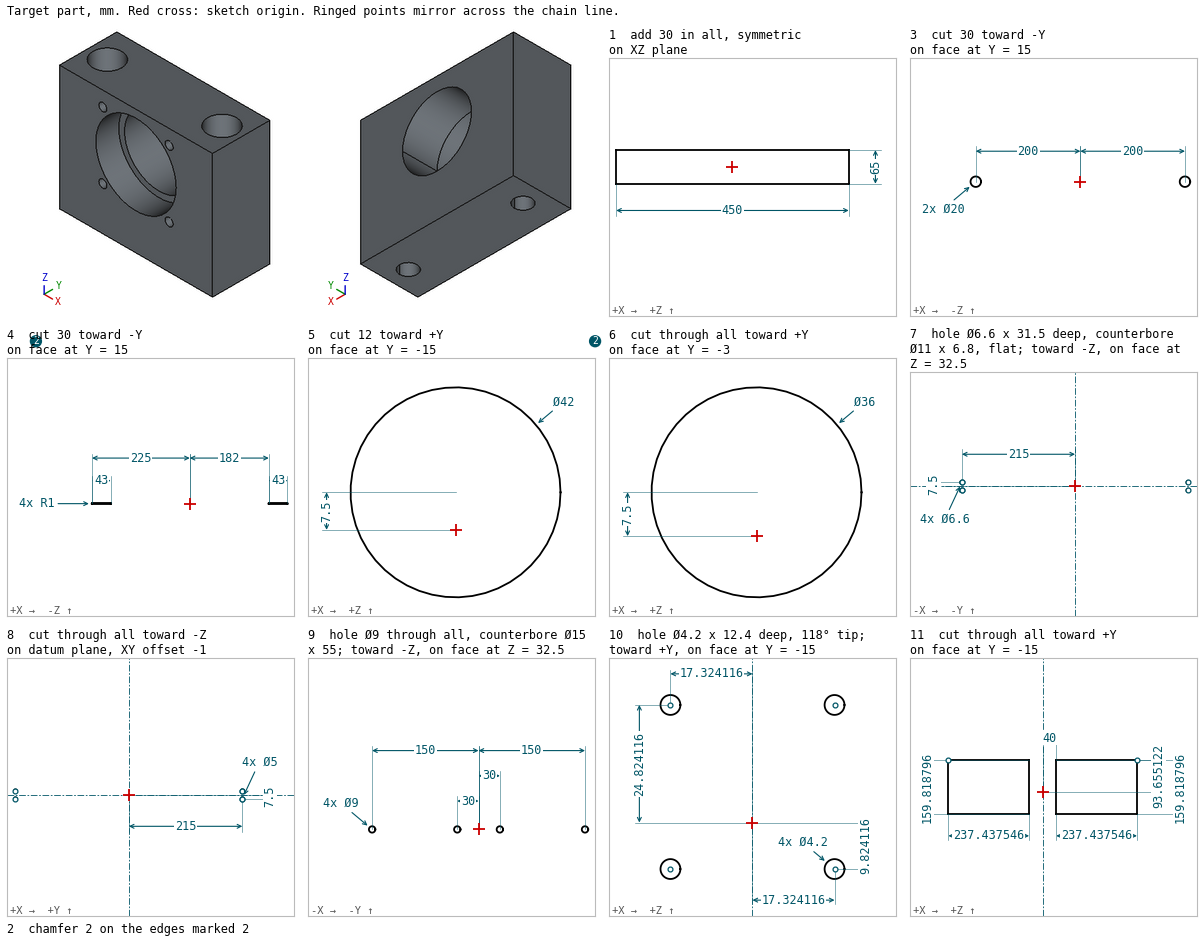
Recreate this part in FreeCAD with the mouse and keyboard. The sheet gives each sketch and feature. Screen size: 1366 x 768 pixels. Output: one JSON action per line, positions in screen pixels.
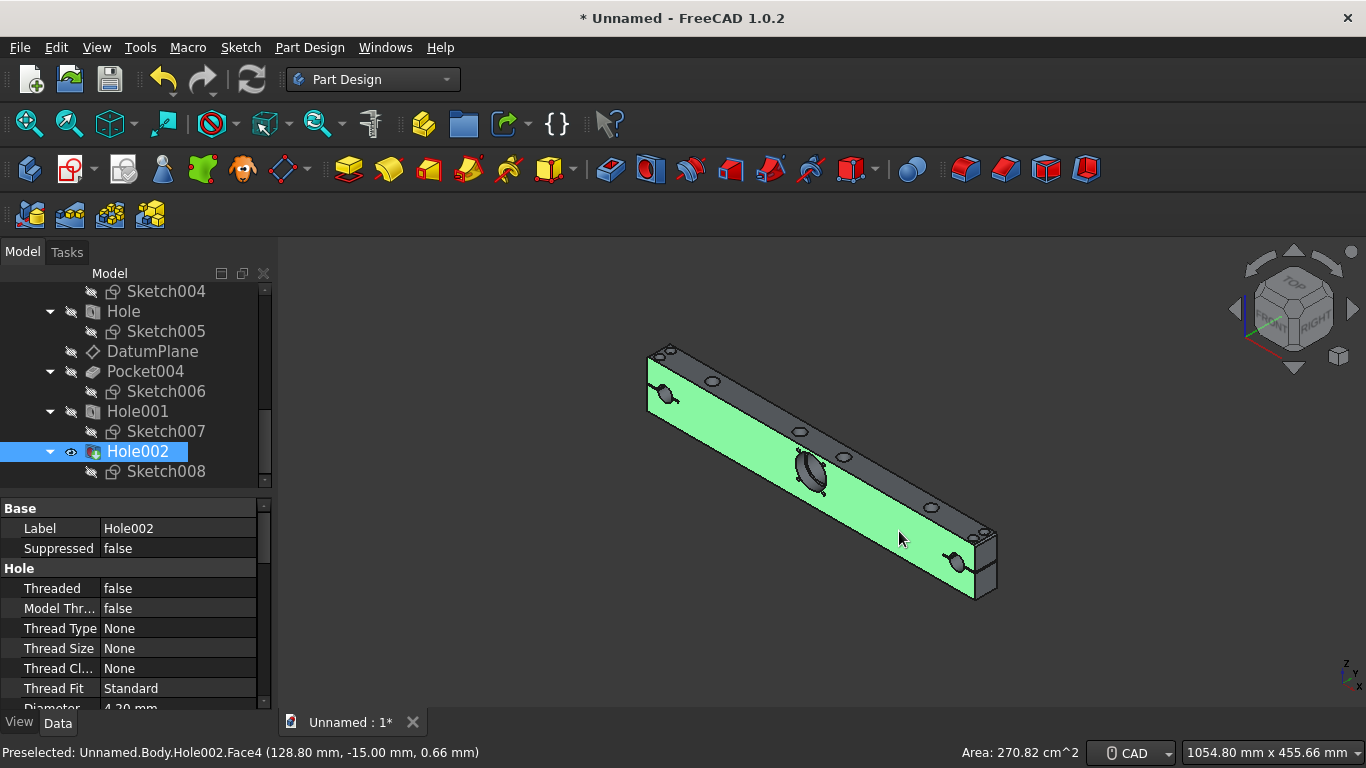
{"action": "left_click", "coordinate": [70, 170]}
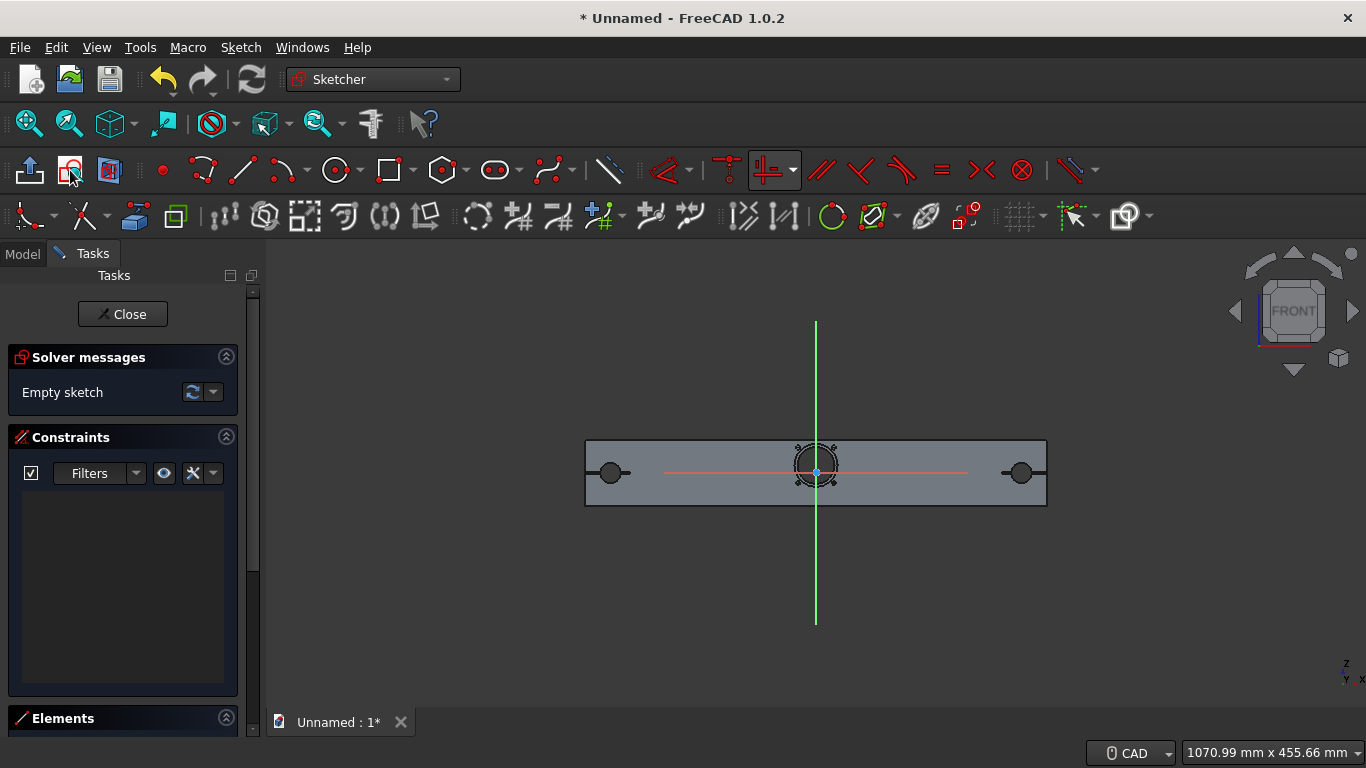
{"action": "key", "text": "g r"}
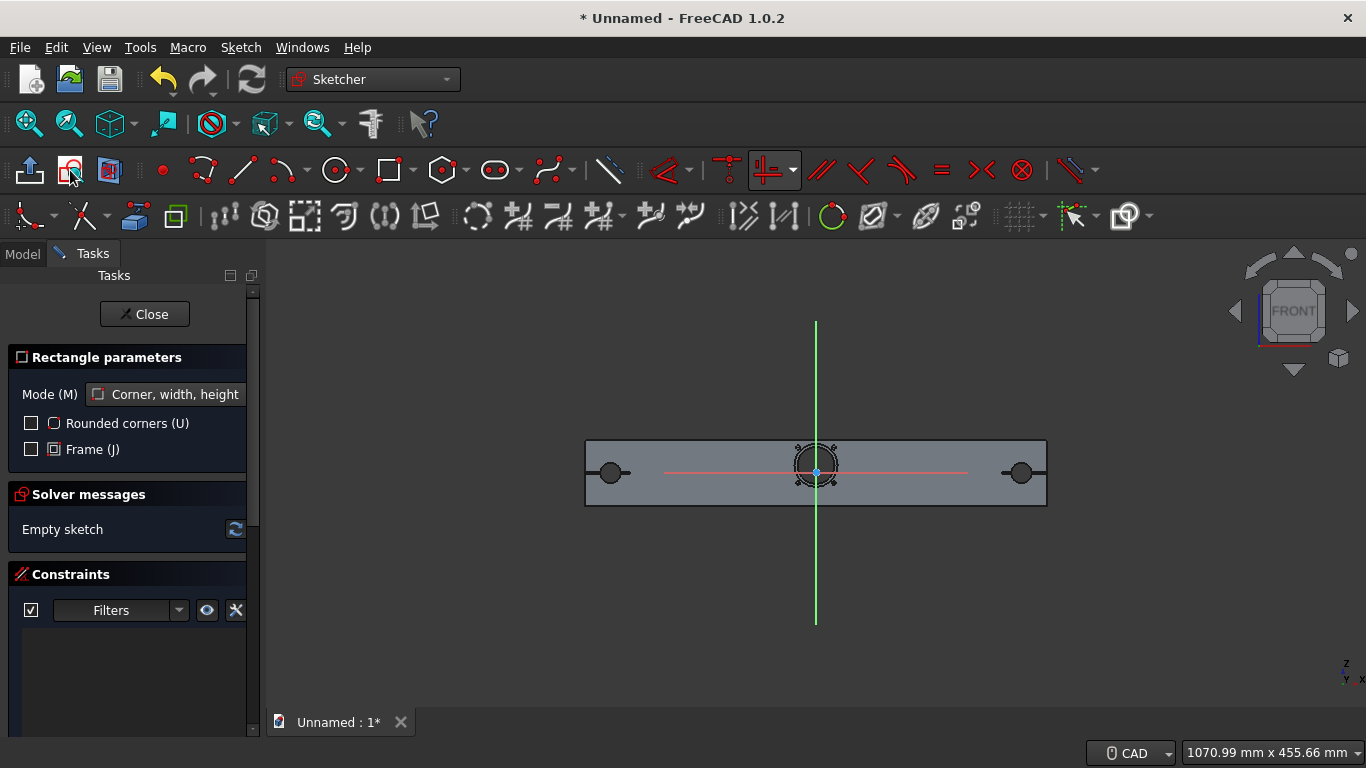
{"action": "left_click", "coordinate": [857, 377]}
{"action": "mouse_move", "coordinate": [1101, 541]}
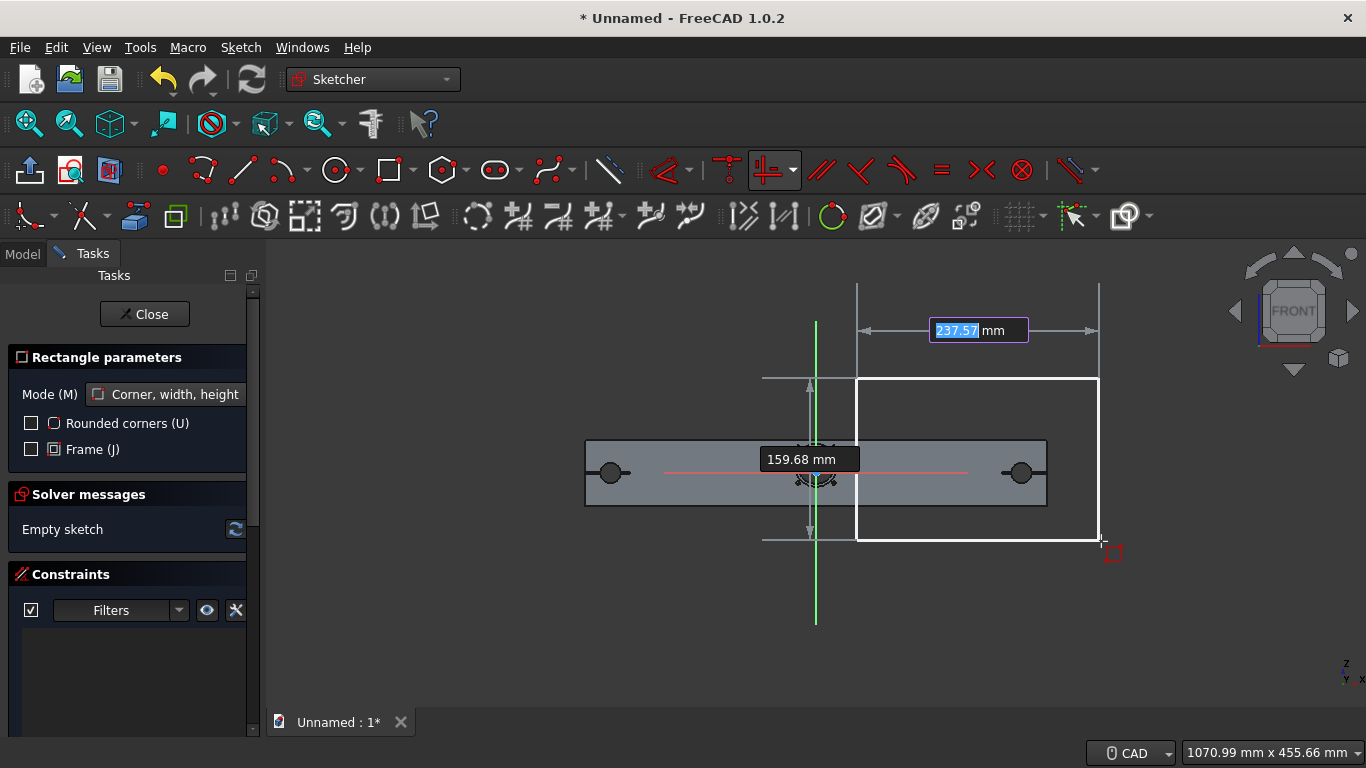
{"action": "type", "text": "237.437546"}
{"action": "key", "text": "Tab"}
{"action": "type", "text": "159.818796"}
{"action": "key", "text": "Return"}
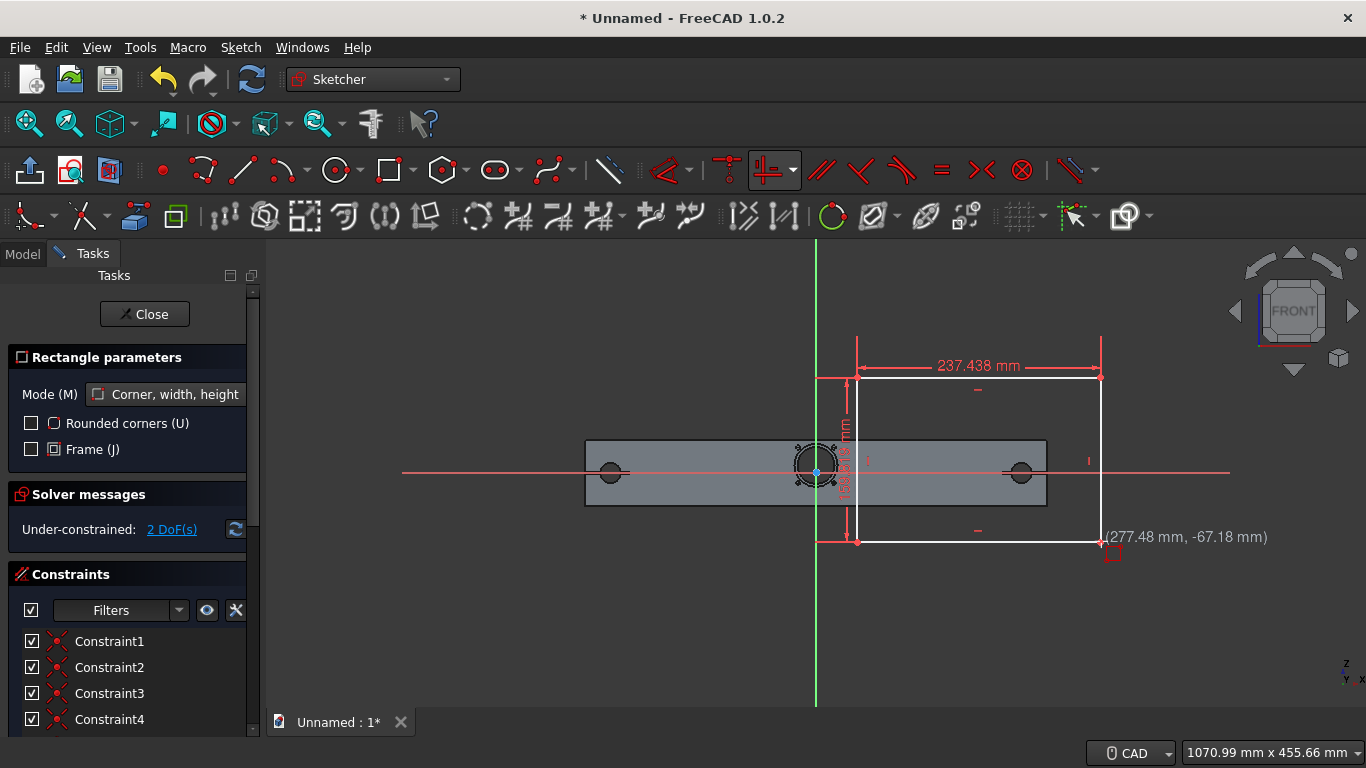
{"action": "left_click", "coordinate": [531, 377]}
{"action": "mouse_move", "coordinate": [775, 541]}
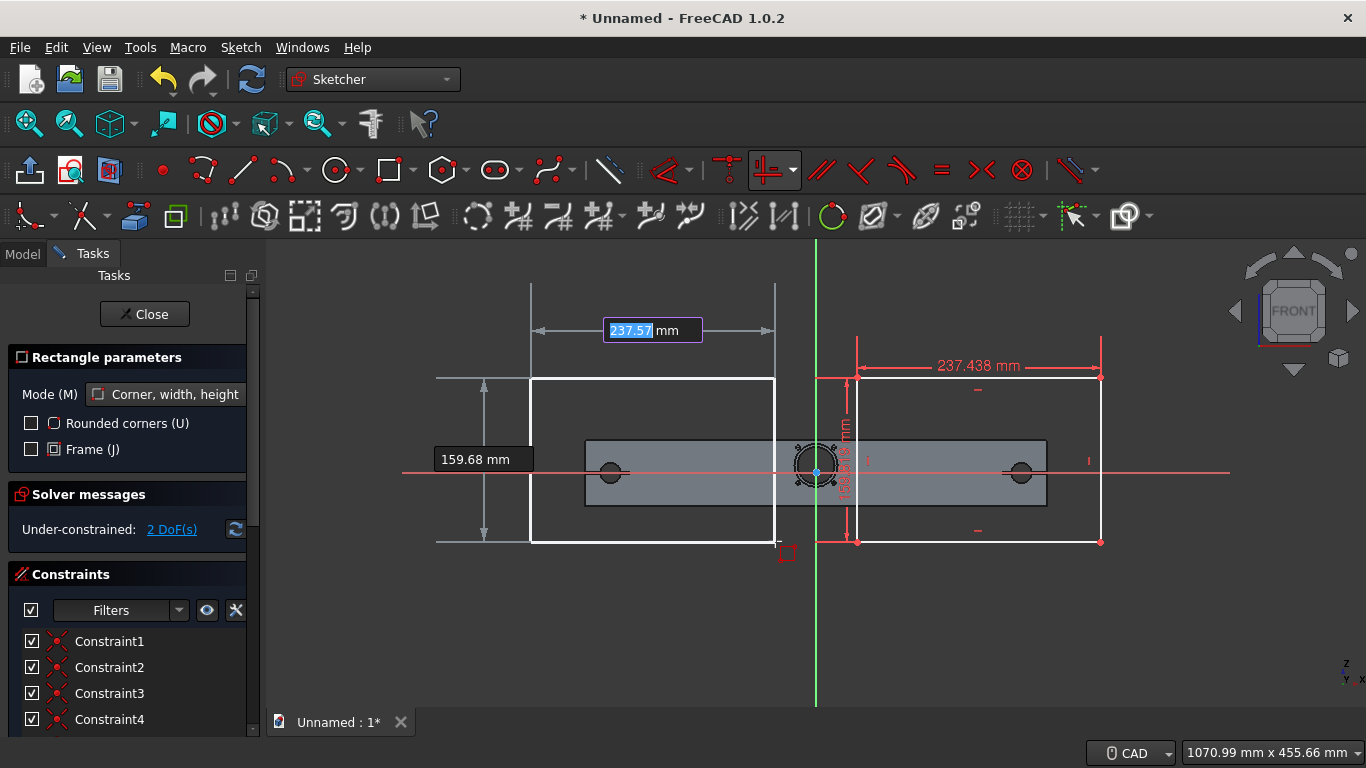
{"action": "type", "text": "237.437546"}
{"action": "key", "text": "Tab"}
{"action": "type", "text": "159.818796"}
{"action": "key", "text": "Return"}
{"action": "key", "text": "Escape"}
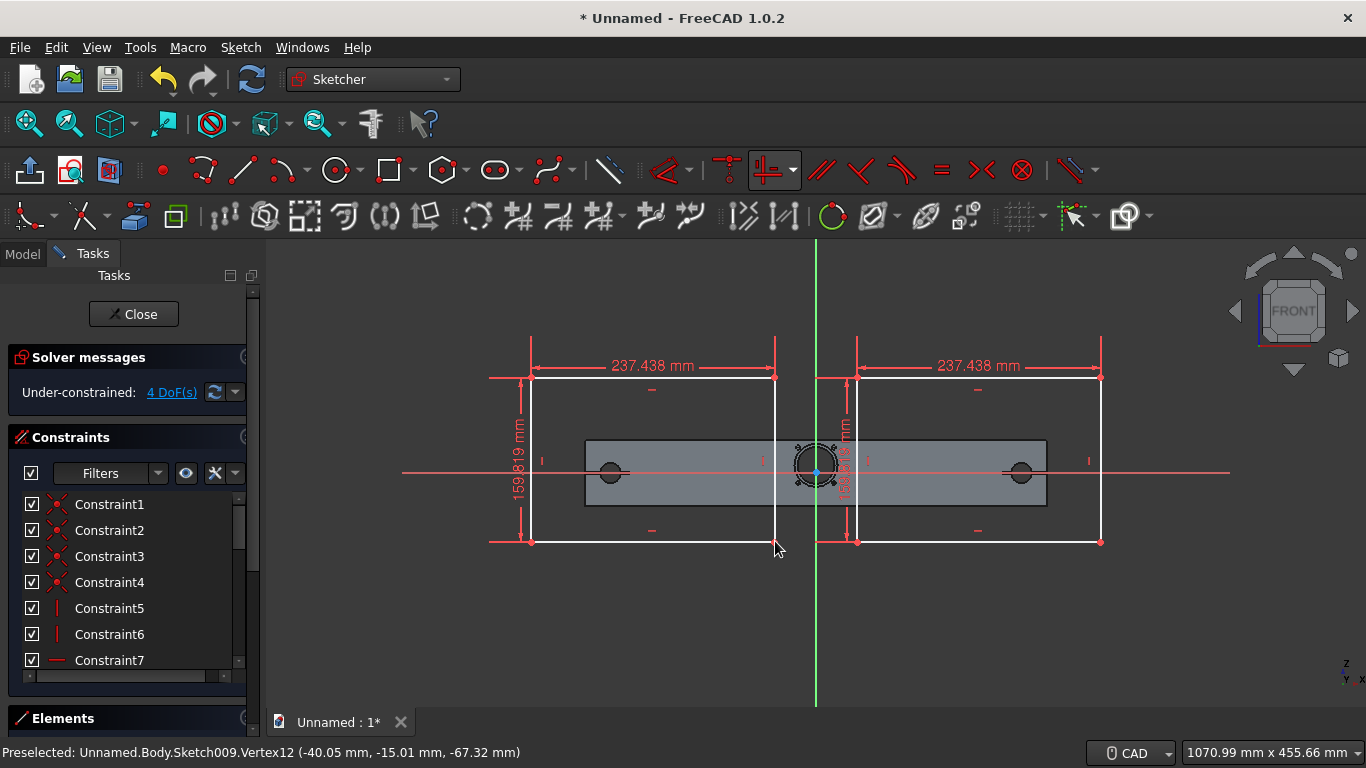
{"action": "left_click", "coordinate": [1101, 378]}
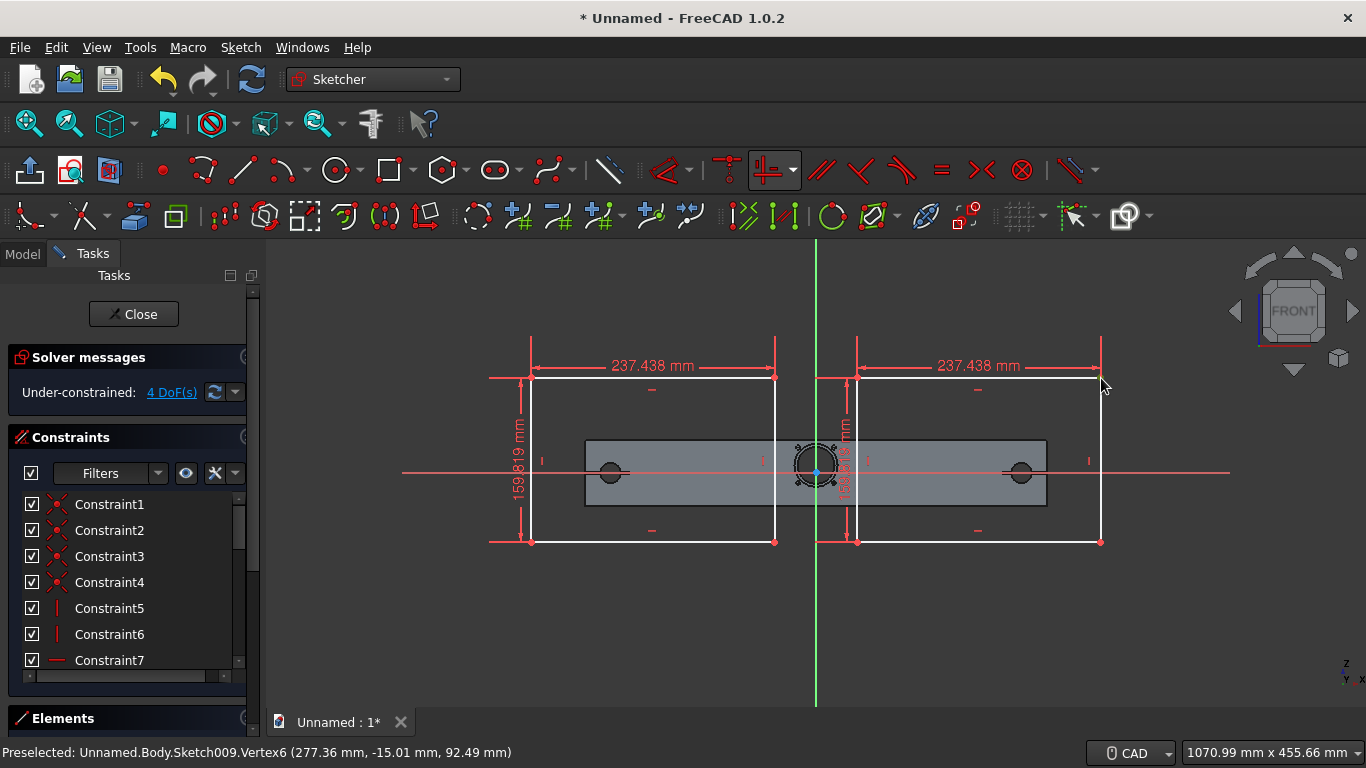
{"action": "left_click", "coordinate": [531, 378]}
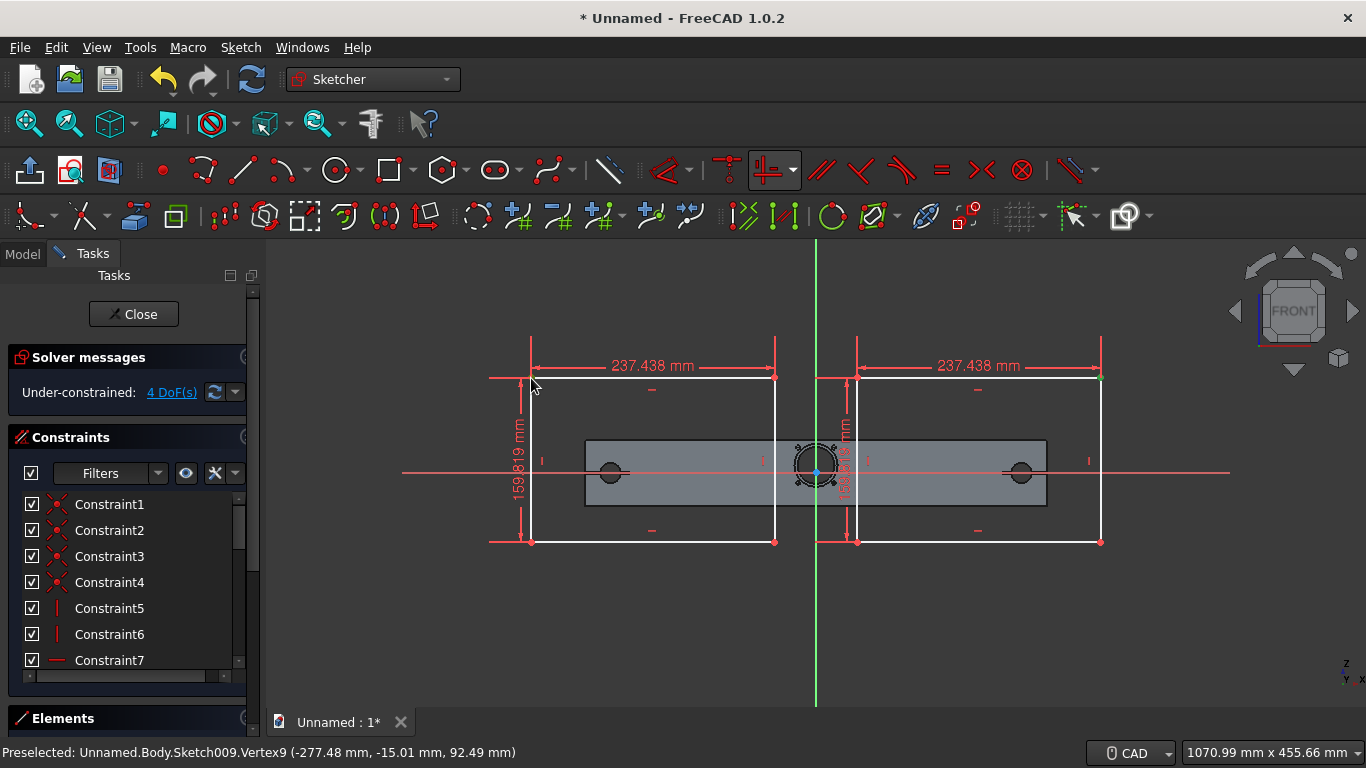
{"action": "left_click", "coordinate": [816, 650]}